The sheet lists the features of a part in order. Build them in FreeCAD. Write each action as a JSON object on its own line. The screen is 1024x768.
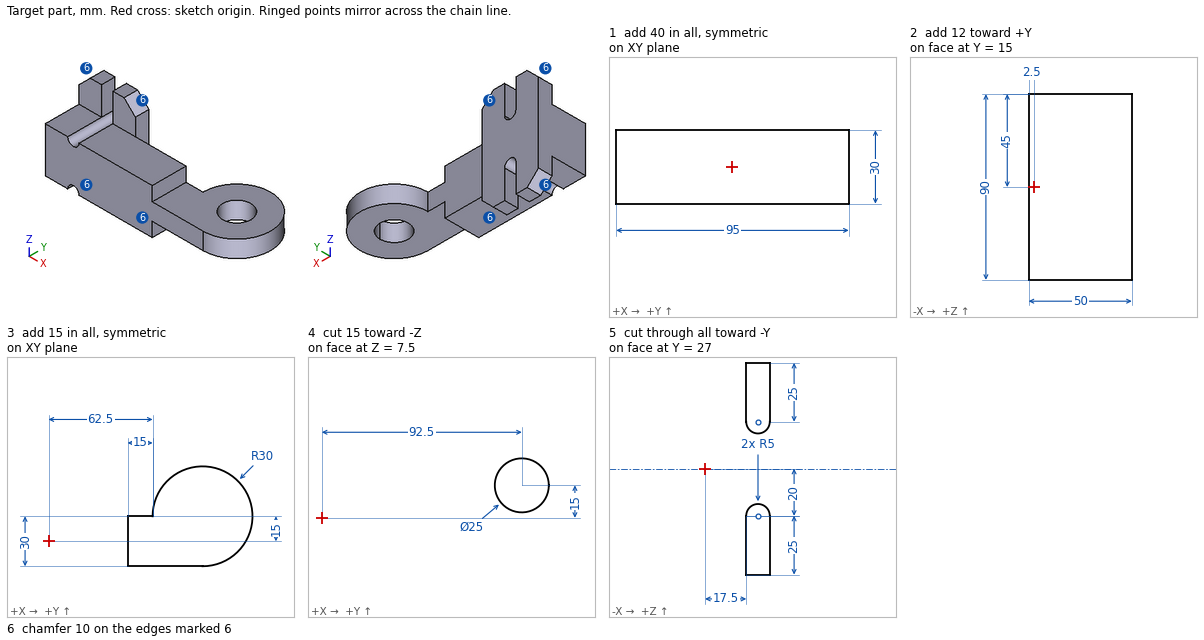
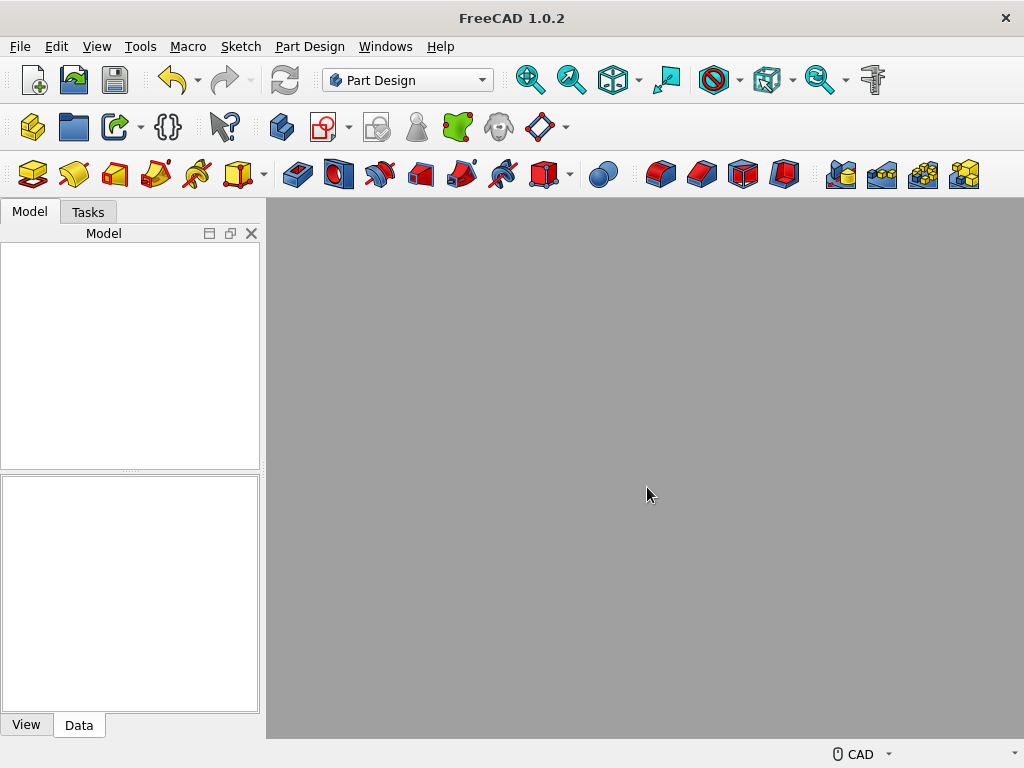
{"action": "left_click", "coordinate": [33, 80]}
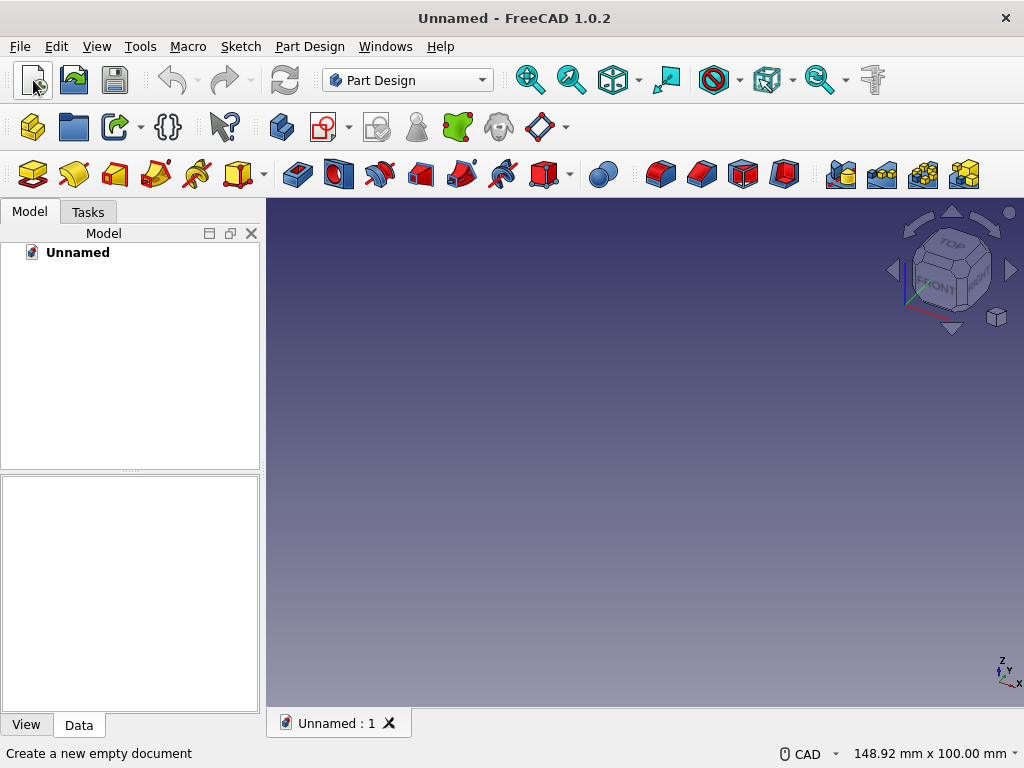
{"action": "left_click", "coordinate": [322, 128]}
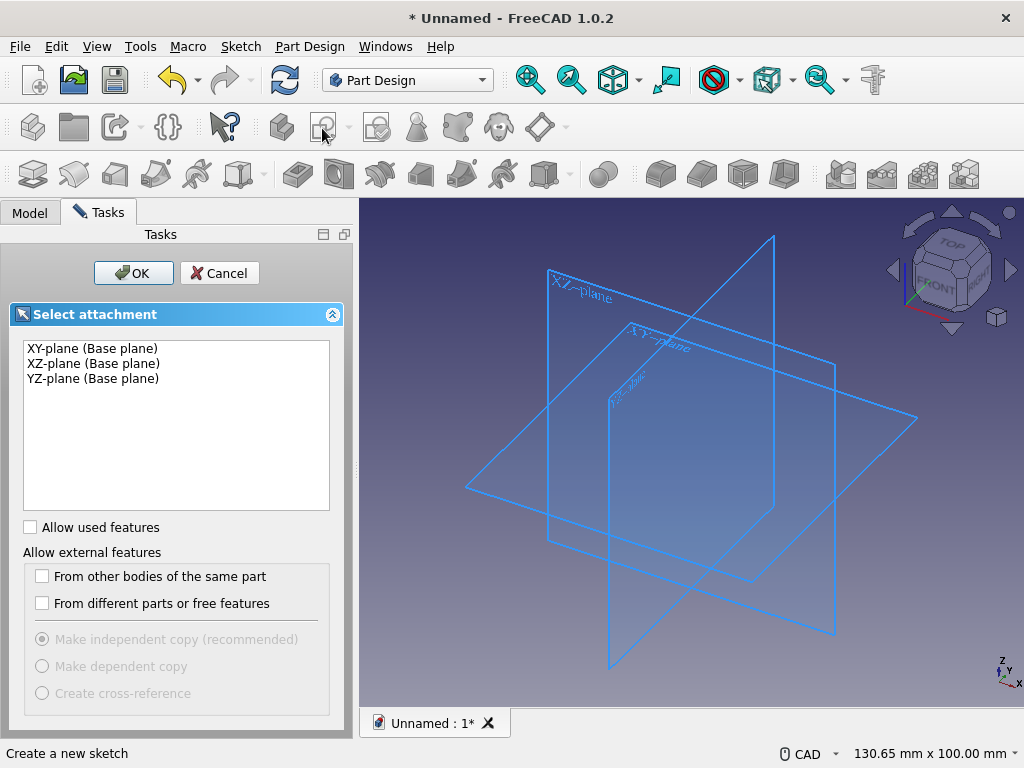
{"action": "left_click", "coordinate": [84, 348]}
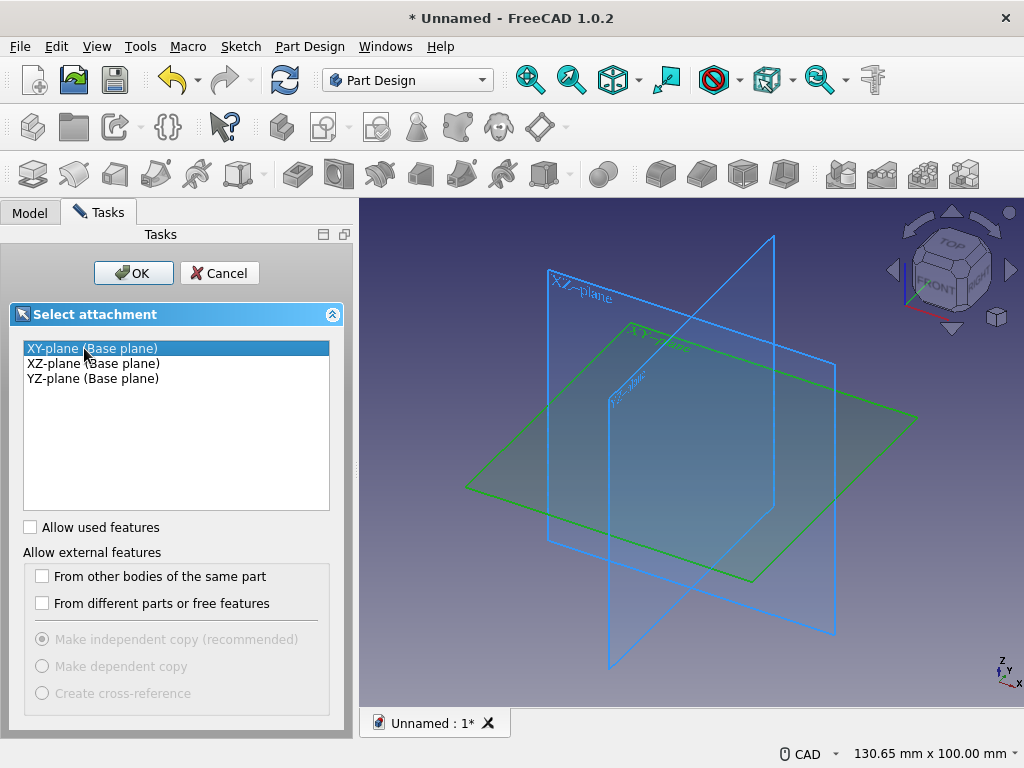
{"action": "left_click", "coordinate": [134, 273]}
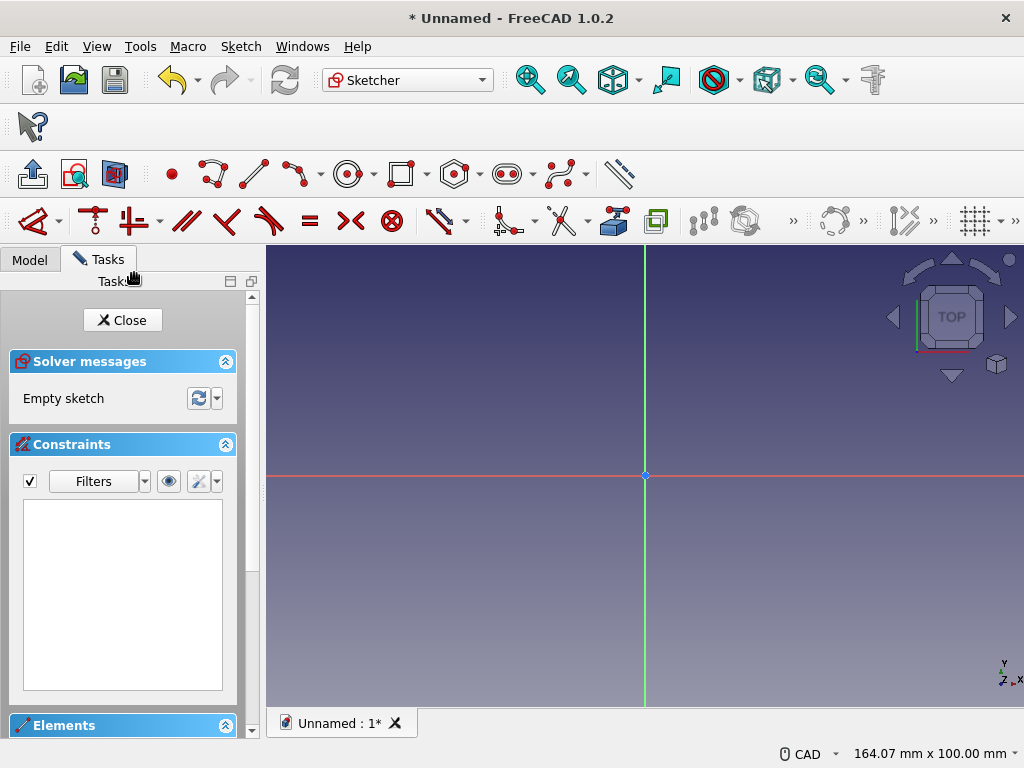
{"action": "scroll", "coordinate": [294, 476], "scroll_direction": "down", "scroll_amount": 1}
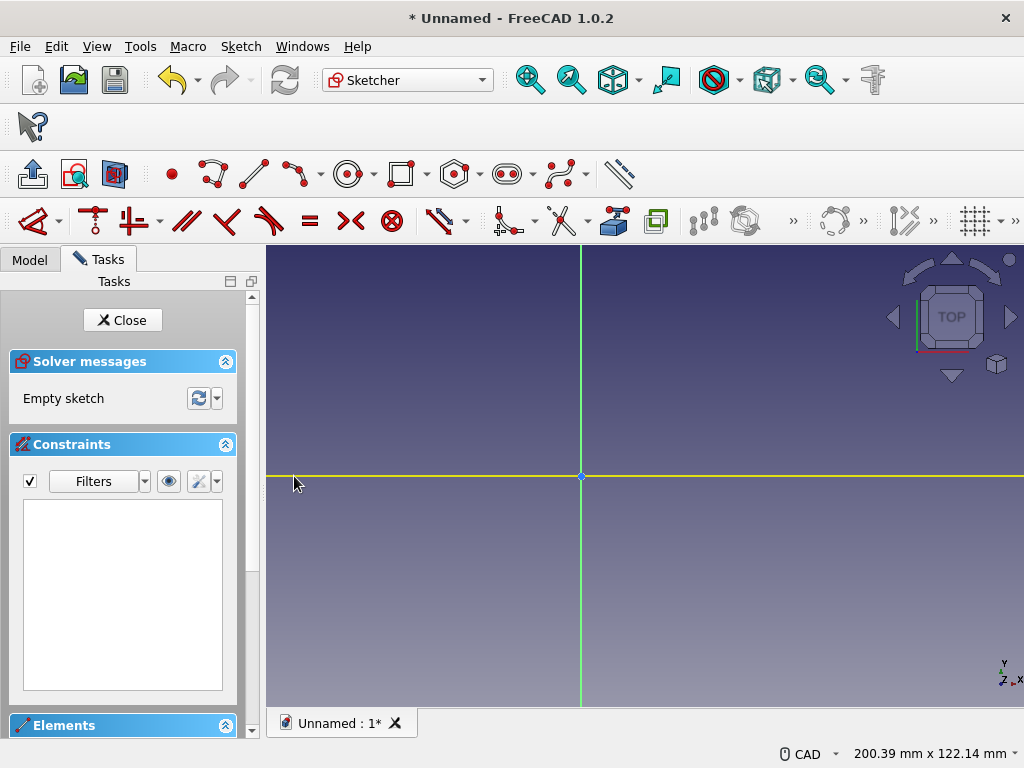
{"action": "key", "text": "g v"}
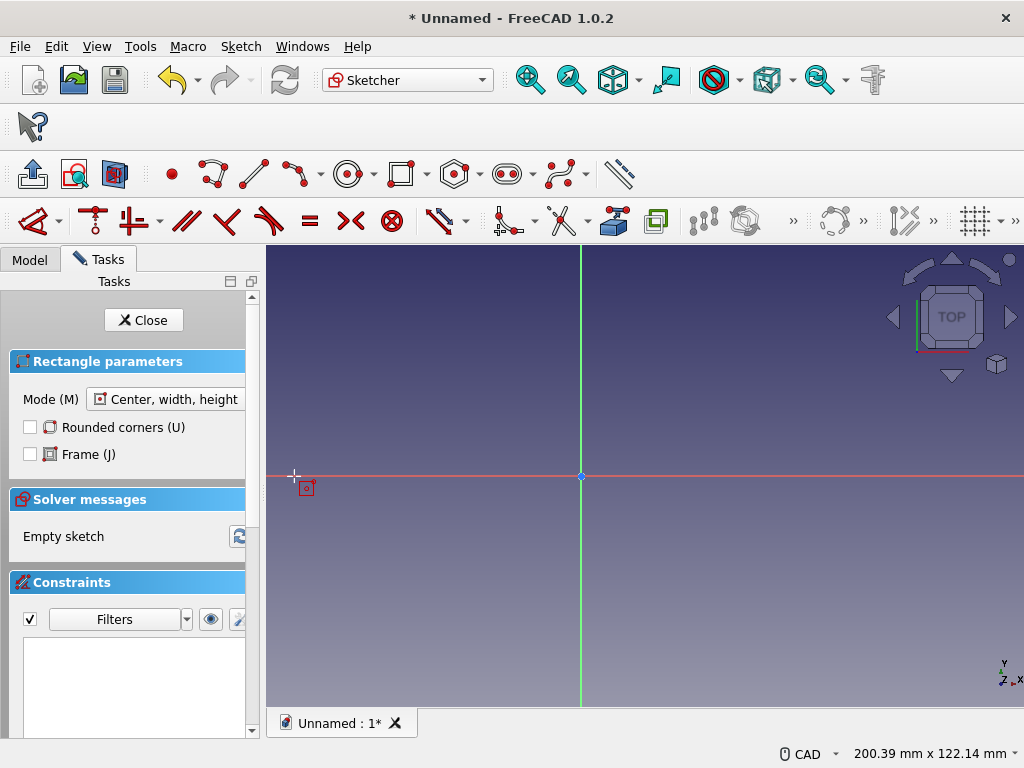
{"action": "left_click", "coordinate": [581, 476]}
{"action": "left_click", "coordinate": [761, 419]}
{"action": "key", "text": "Escape"}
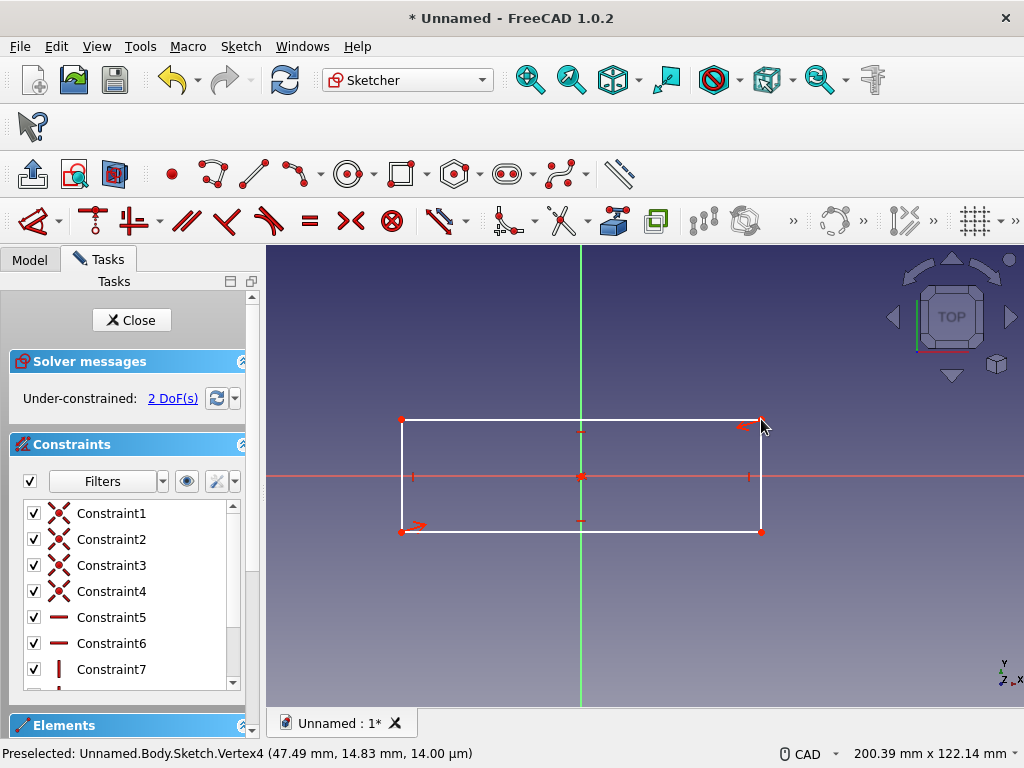
{"action": "left_click", "coordinate": [32, 222]}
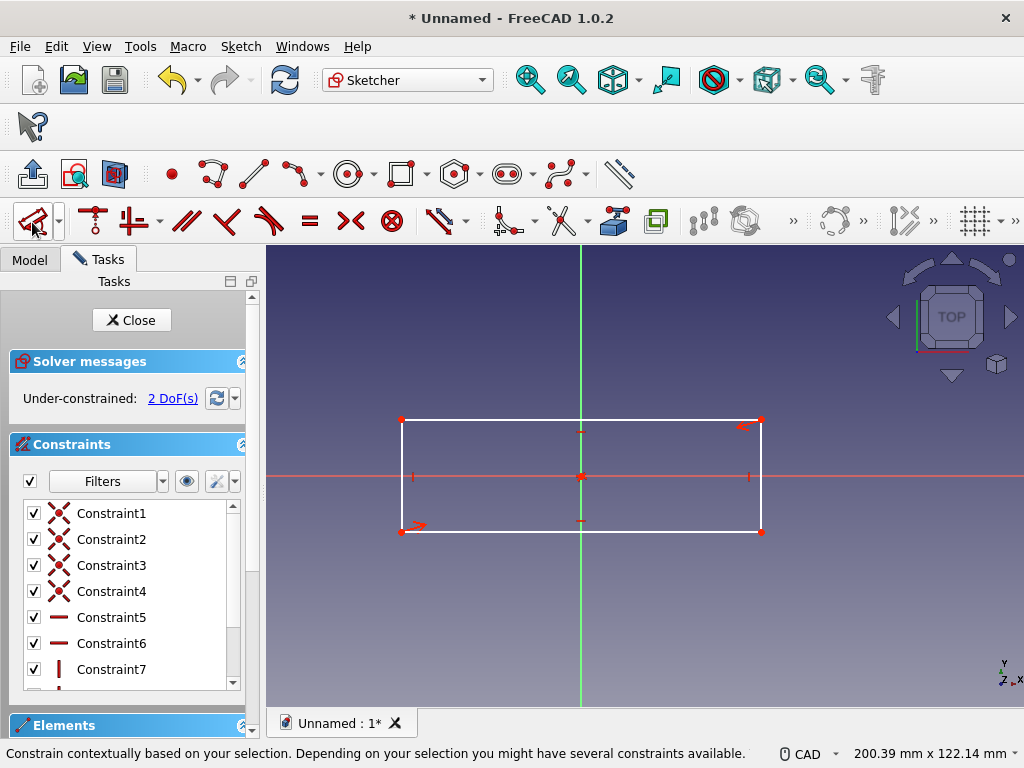
{"action": "left_click", "coordinate": [510, 532]}
{"action": "left_click", "coordinate": [499, 566]}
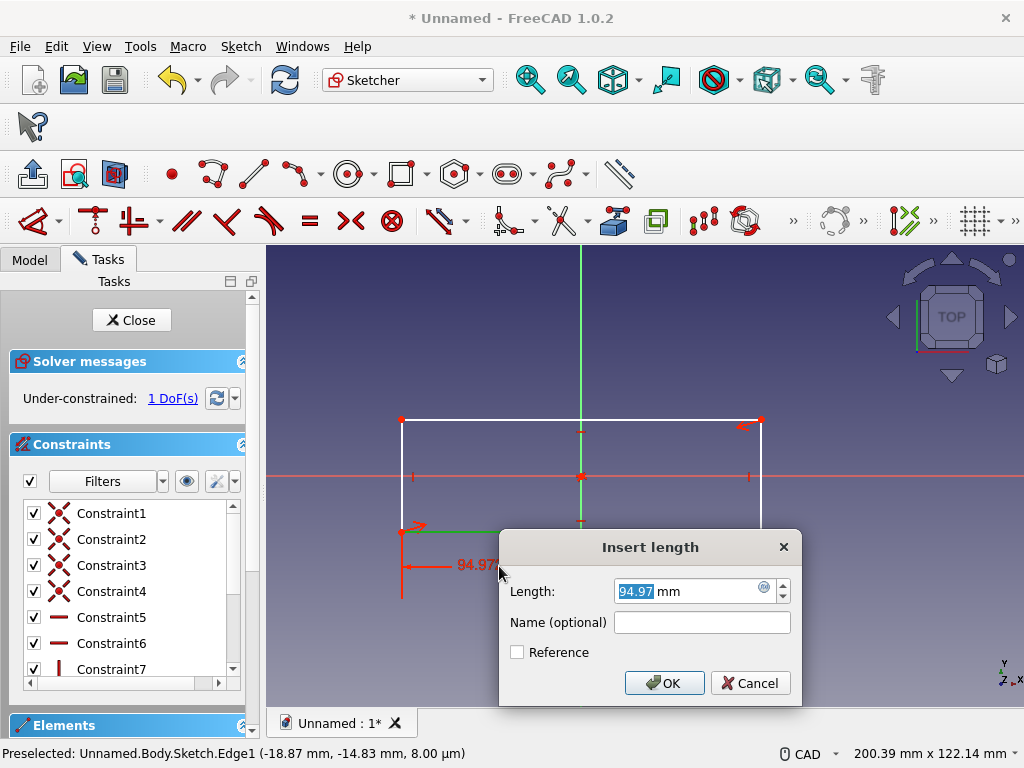
{"action": "type", "text": "95"}
{"action": "key", "text": "Return"}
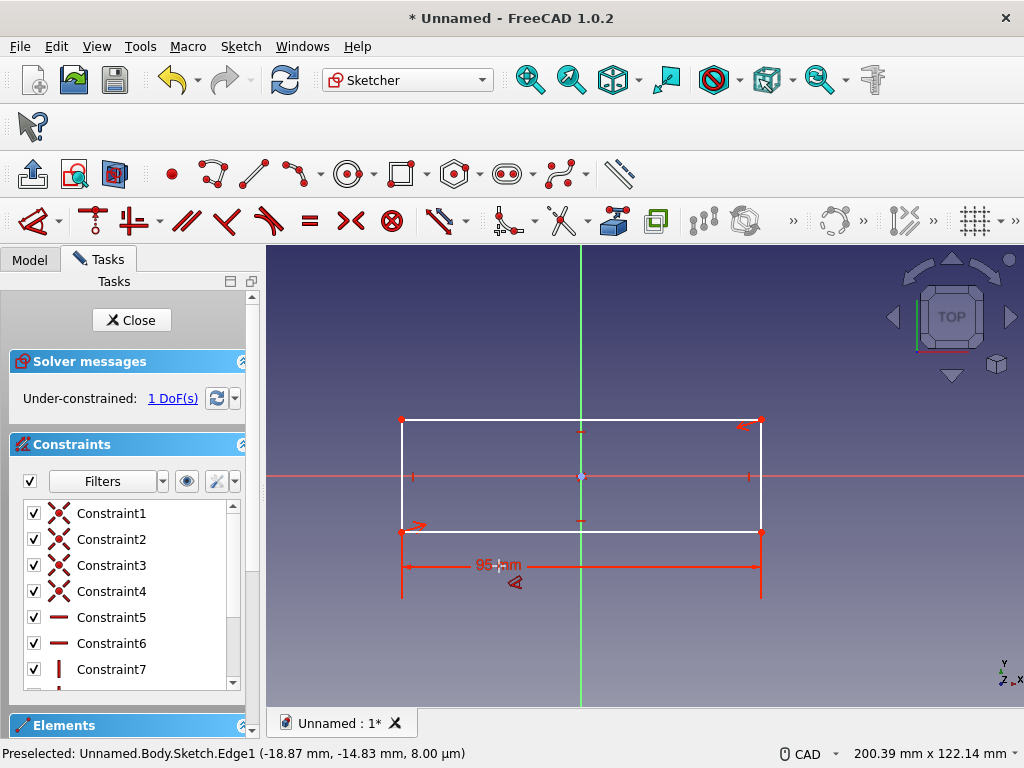
{"action": "left_click", "coordinate": [761, 499]}
{"action": "left_click", "coordinate": [795, 450]}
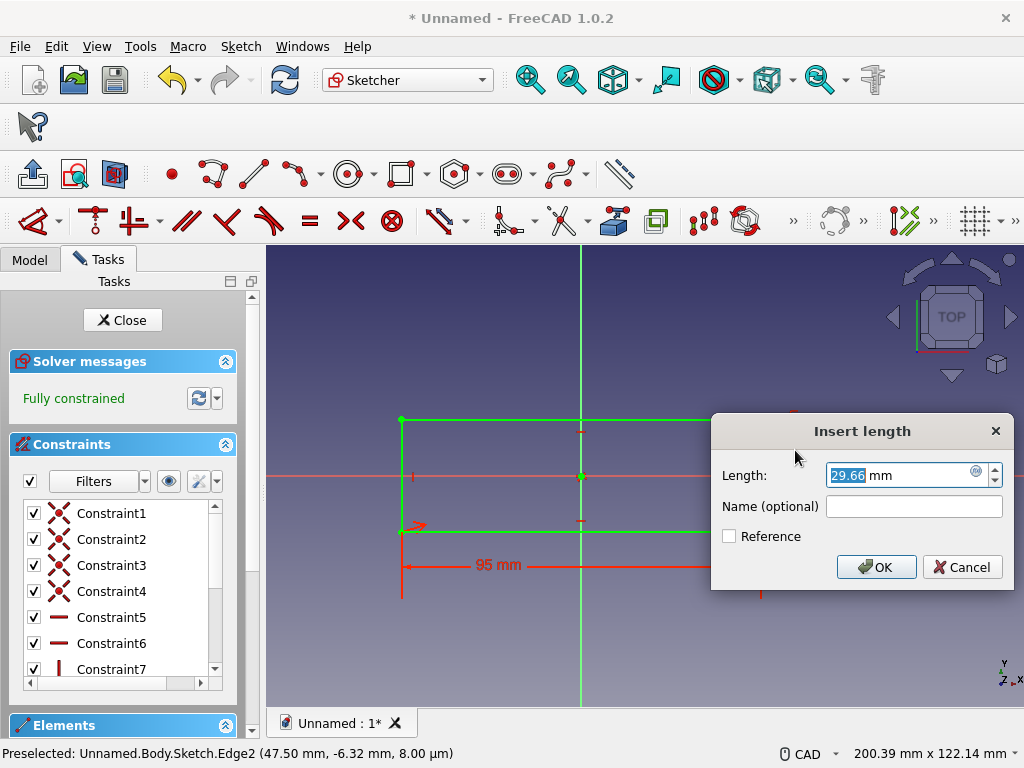
{"action": "type", "text": "30"}
{"action": "key", "text": "Return"}
{"action": "key", "text": "Escape"}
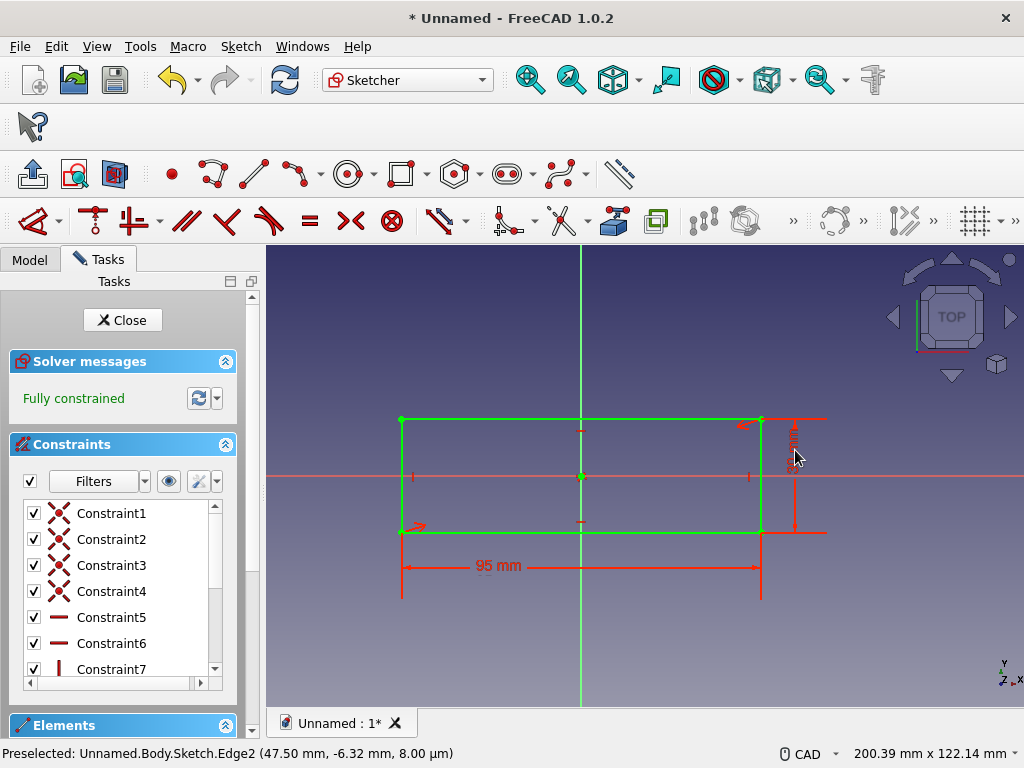
{"action": "left_click", "coordinate": [123, 320]}